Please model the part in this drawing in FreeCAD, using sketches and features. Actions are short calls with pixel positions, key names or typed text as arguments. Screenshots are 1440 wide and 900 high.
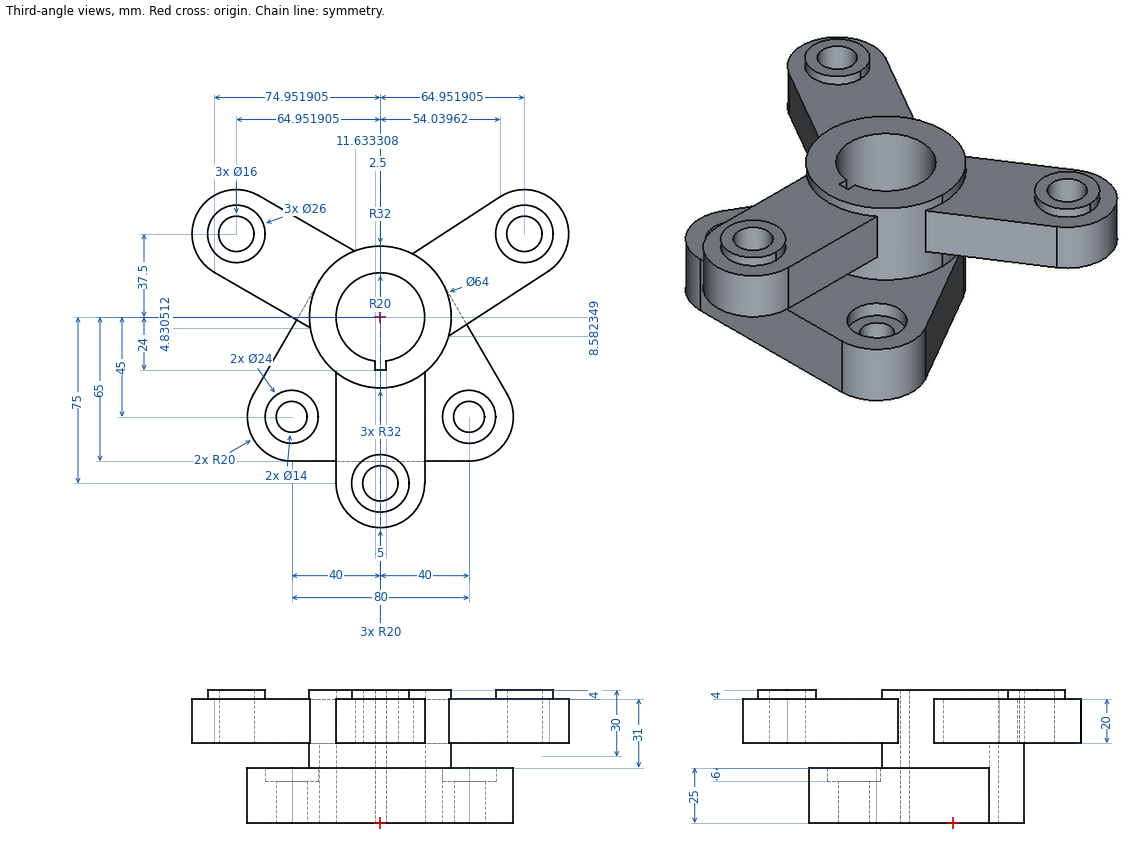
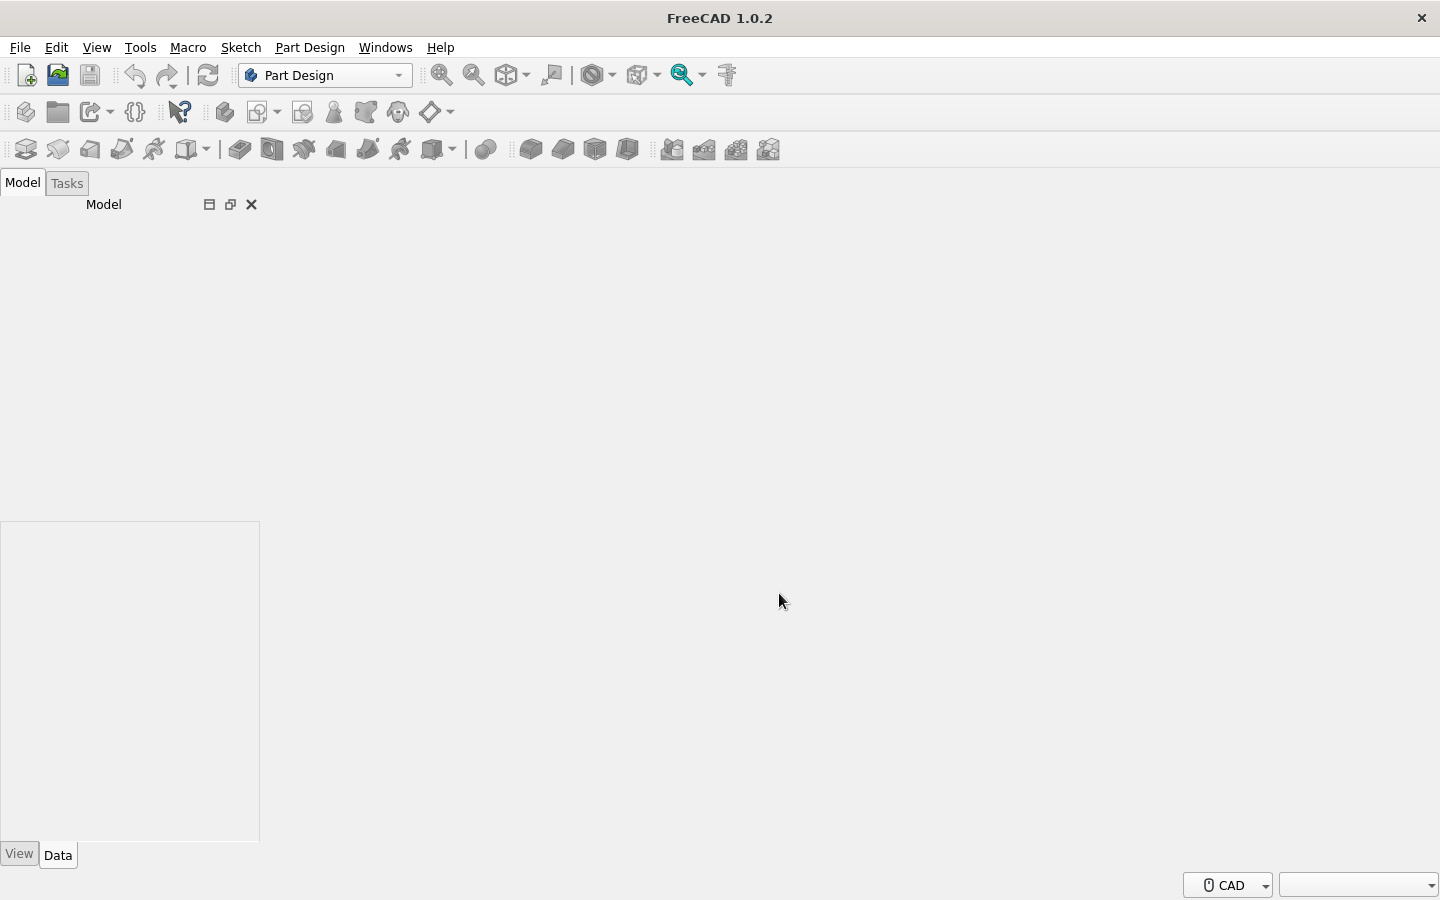
click(26, 76)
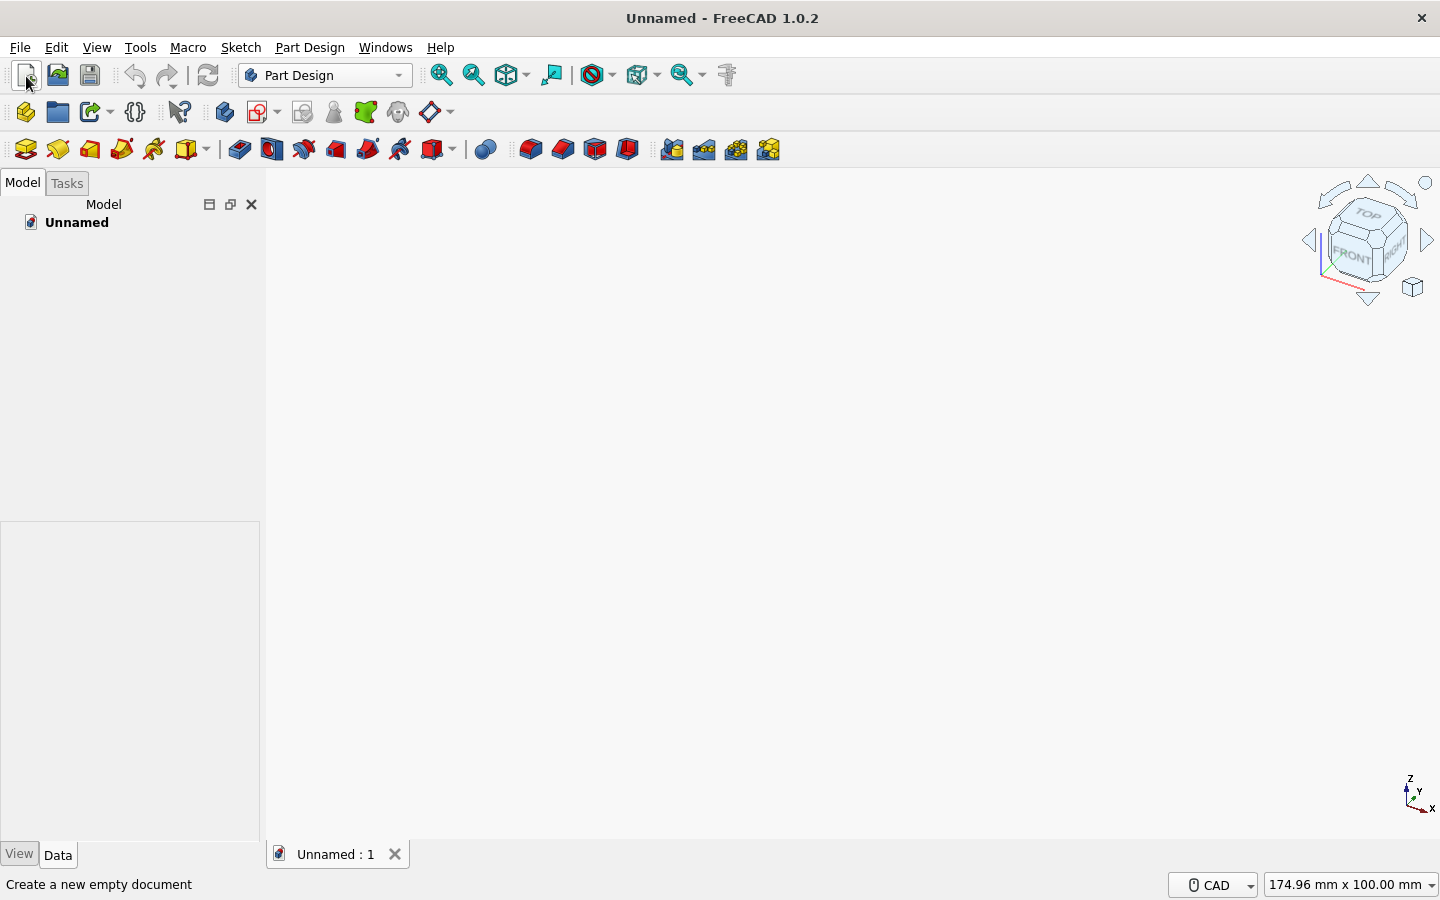
click(258, 112)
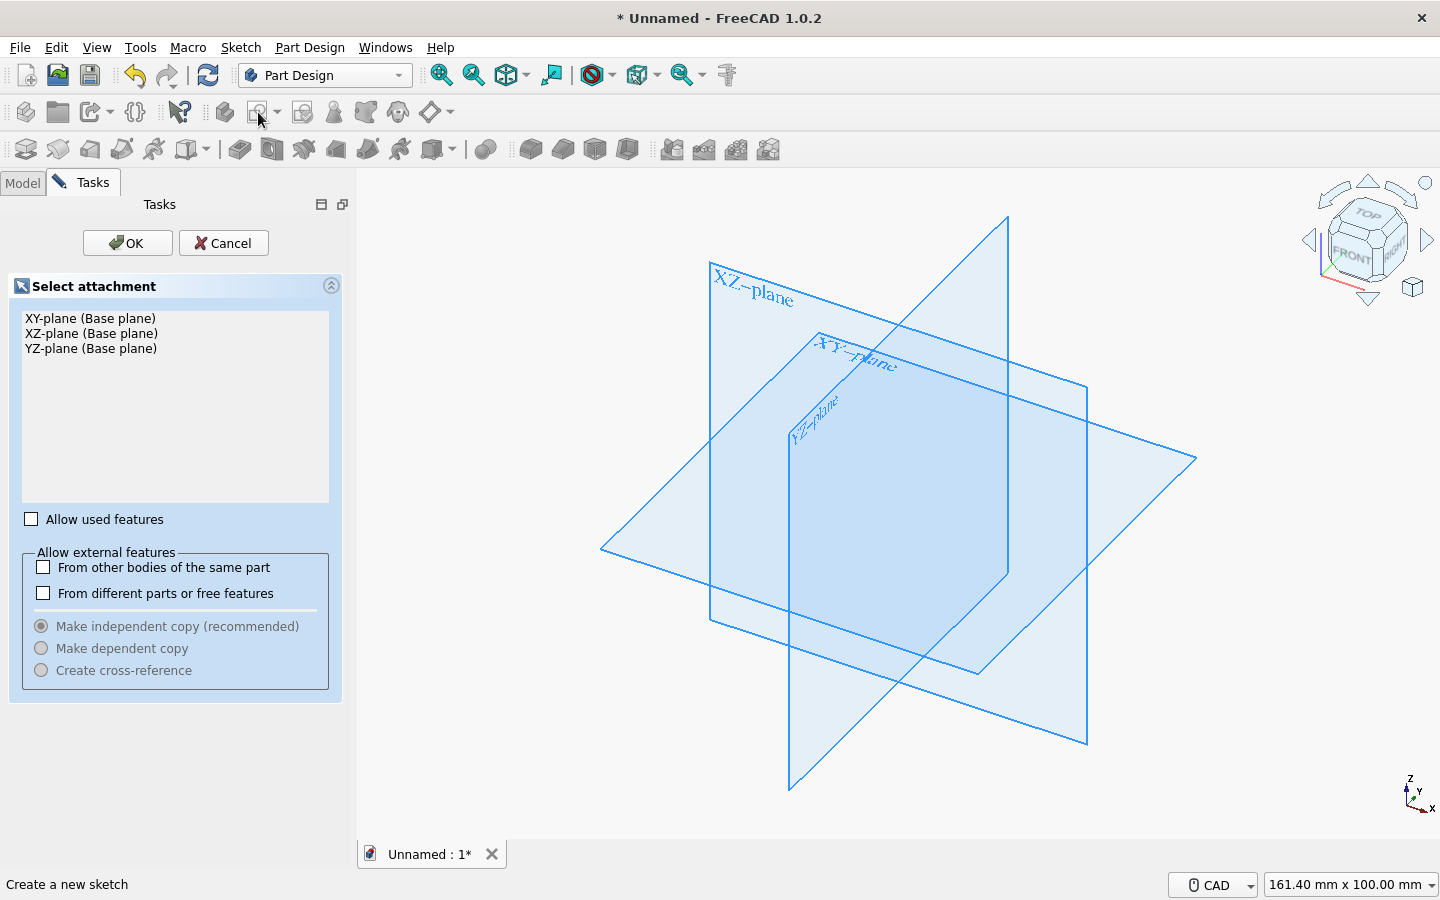
click(82, 318)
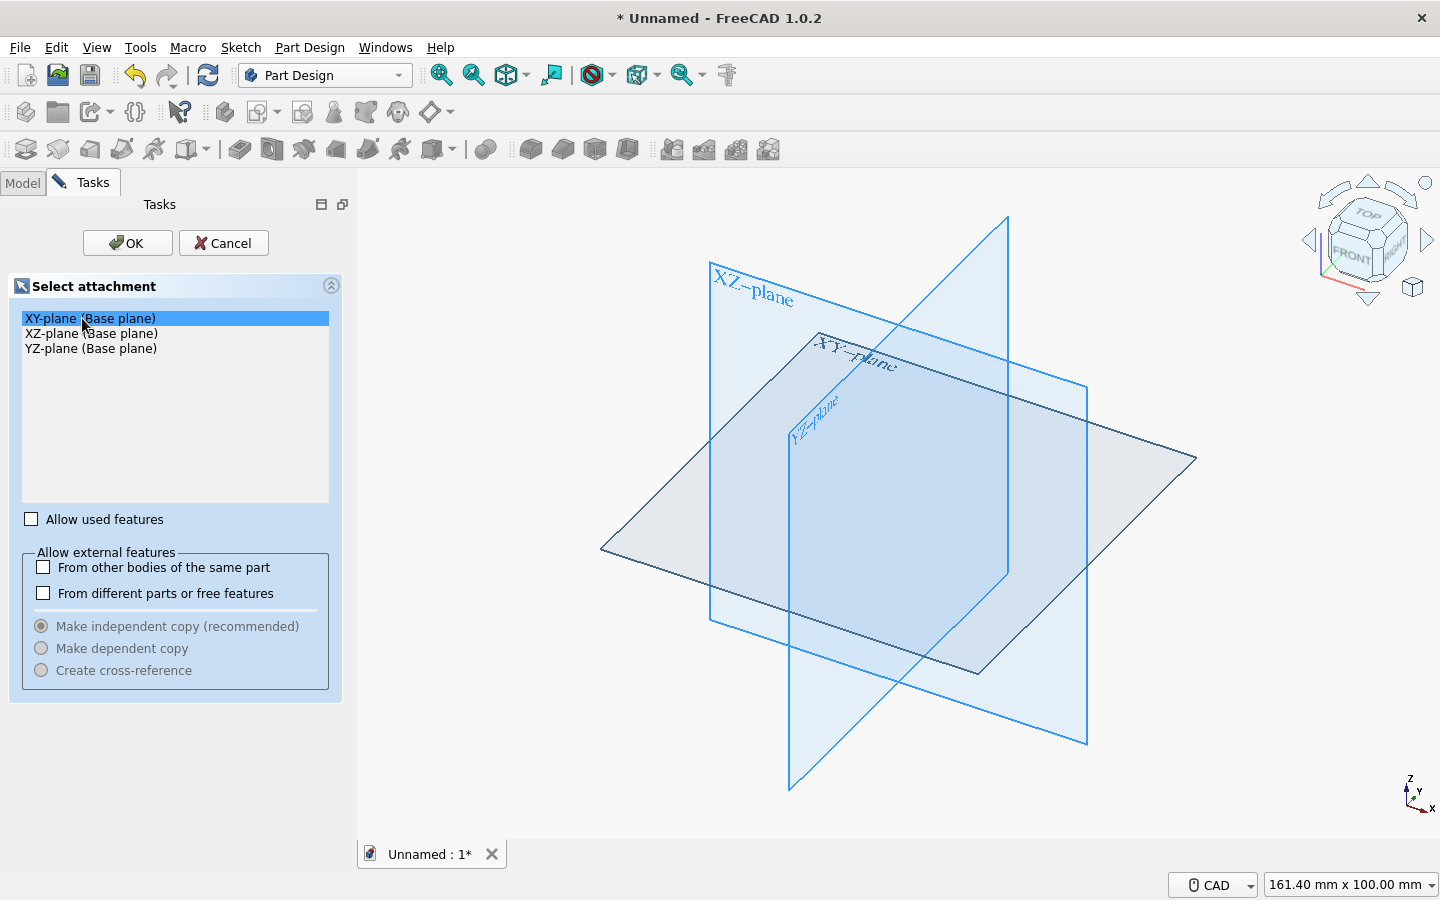
click(128, 243)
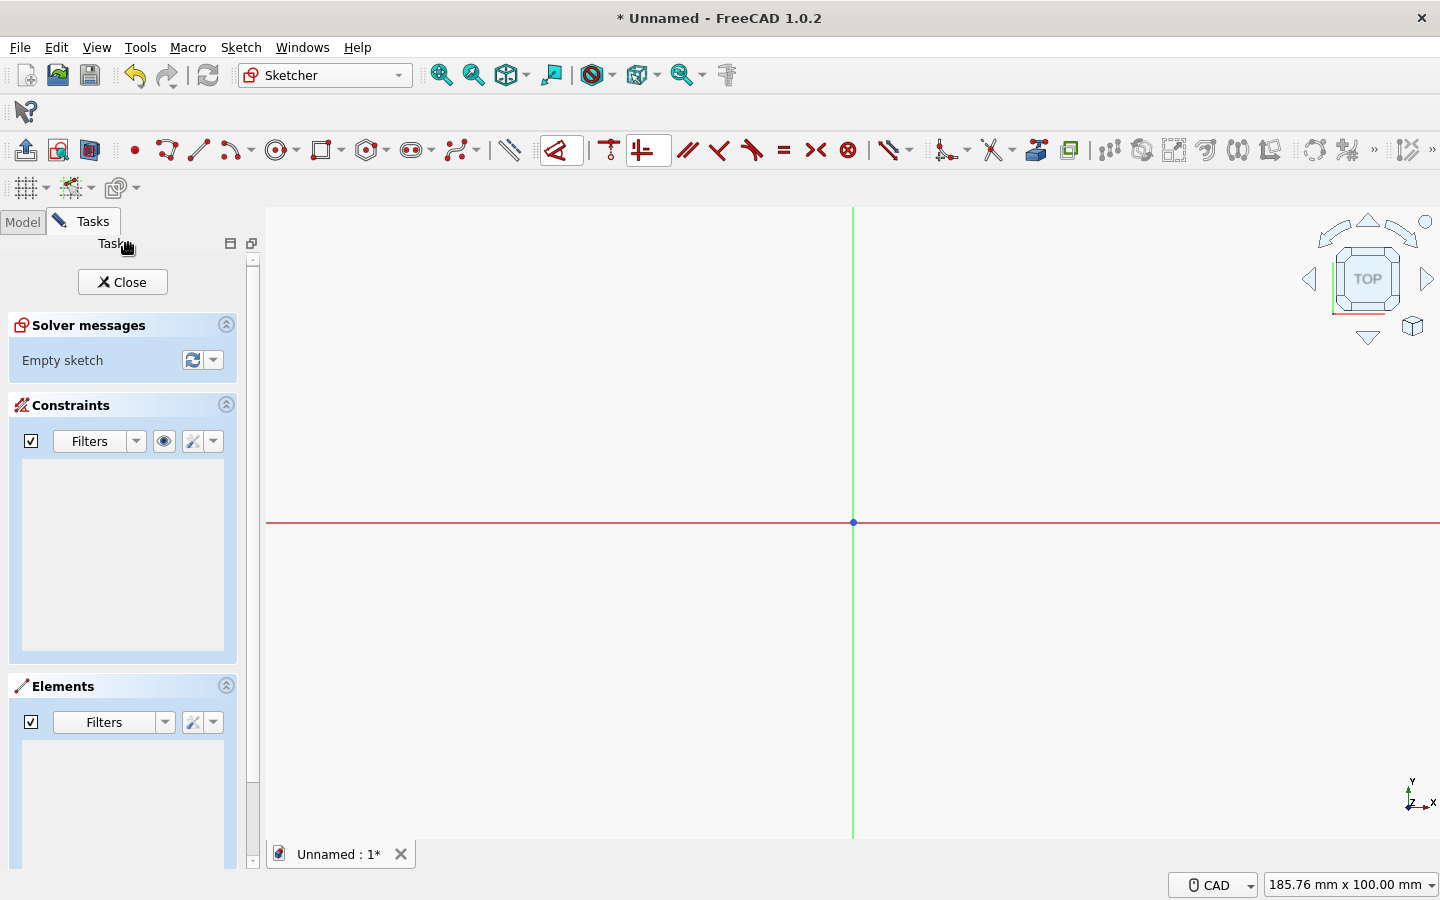
scroll(645, 311, down, 2)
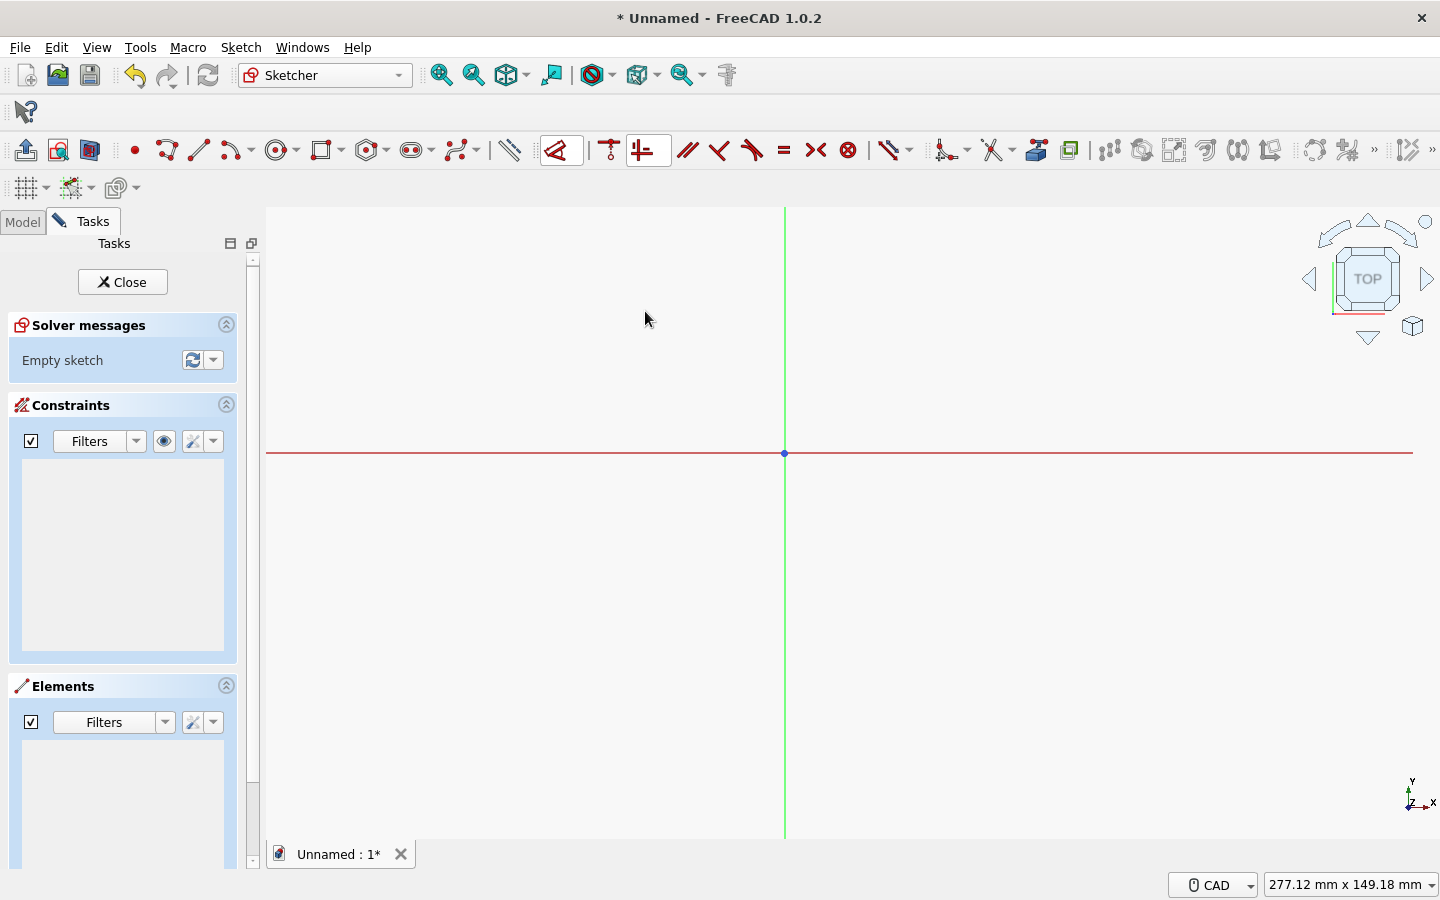
click(200, 150)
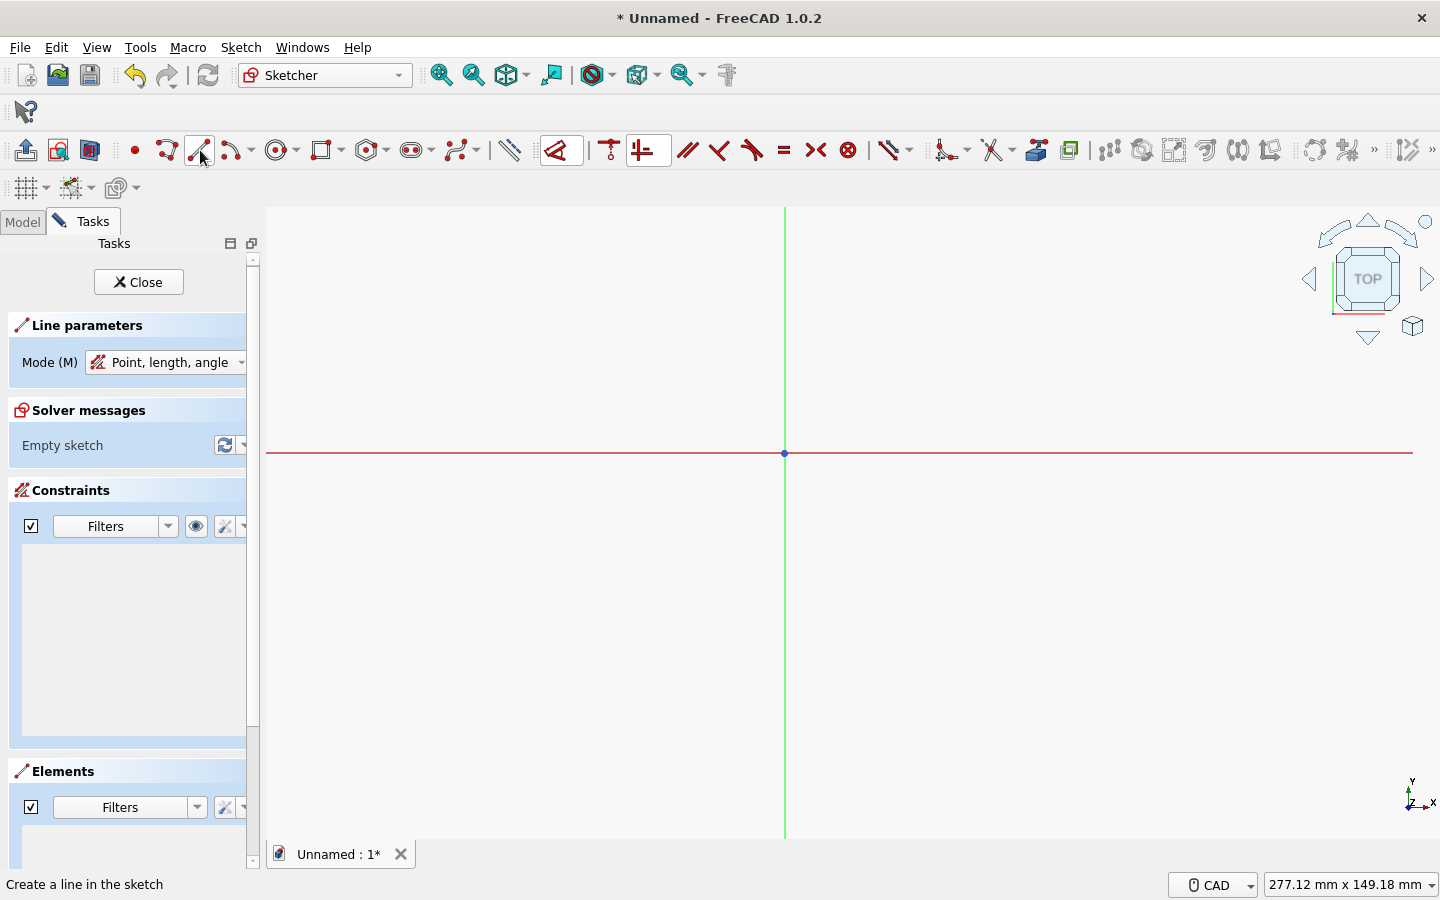
click(667, 385)
click(542, 601)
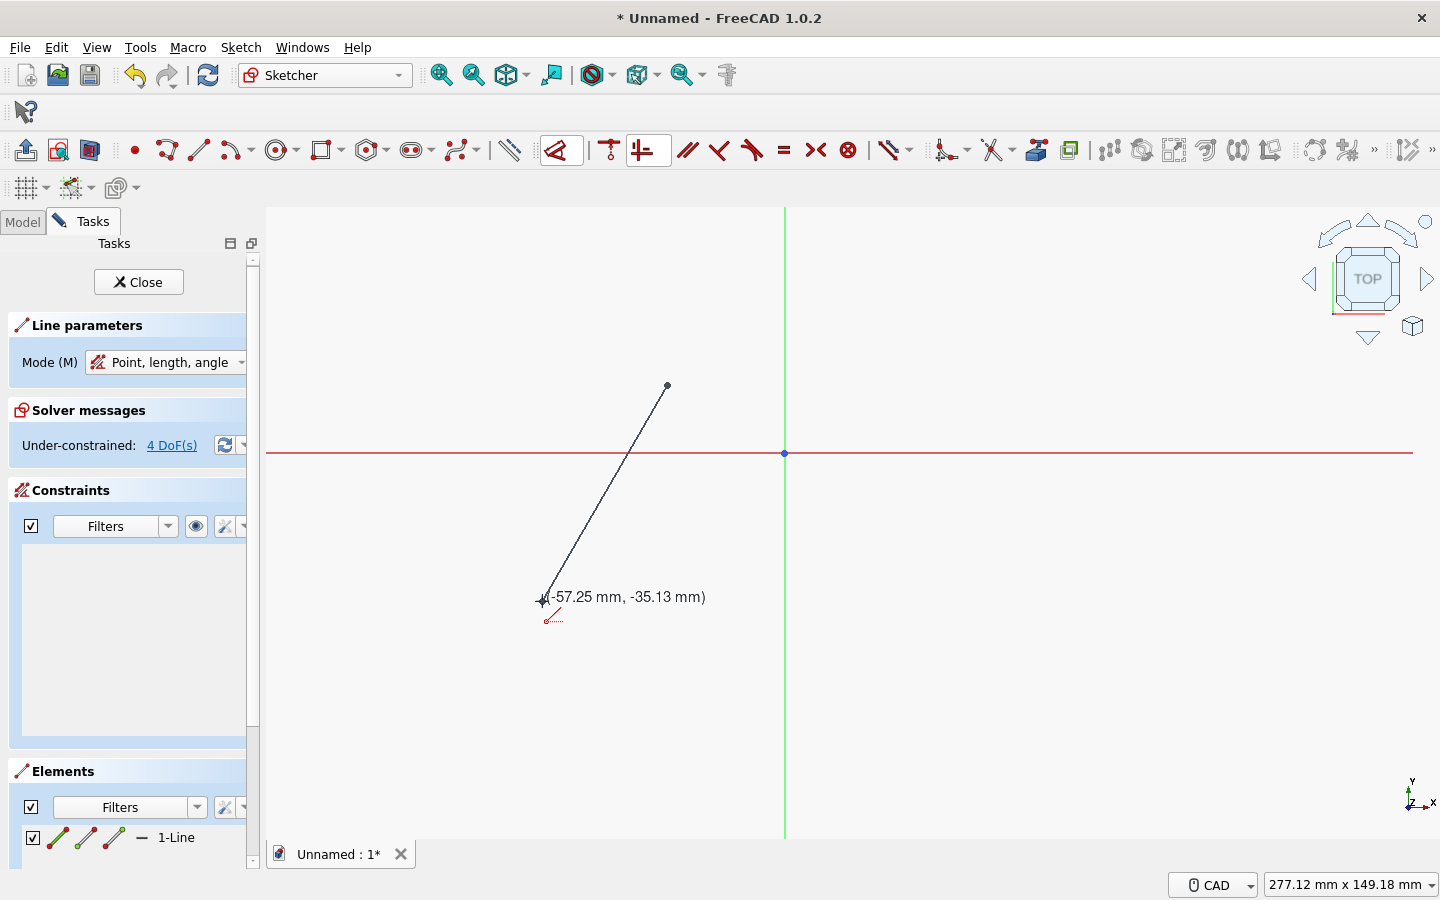
click(615, 729)
click(954, 729)